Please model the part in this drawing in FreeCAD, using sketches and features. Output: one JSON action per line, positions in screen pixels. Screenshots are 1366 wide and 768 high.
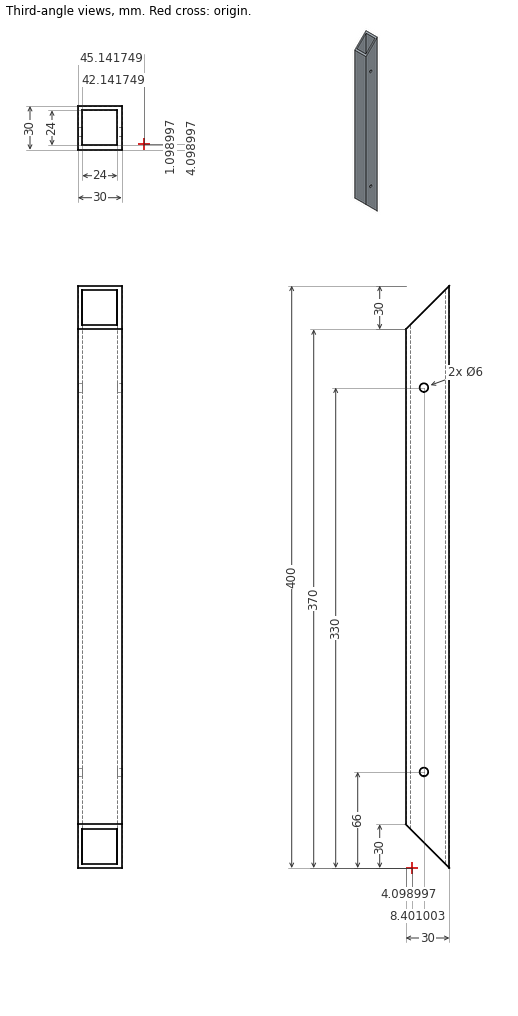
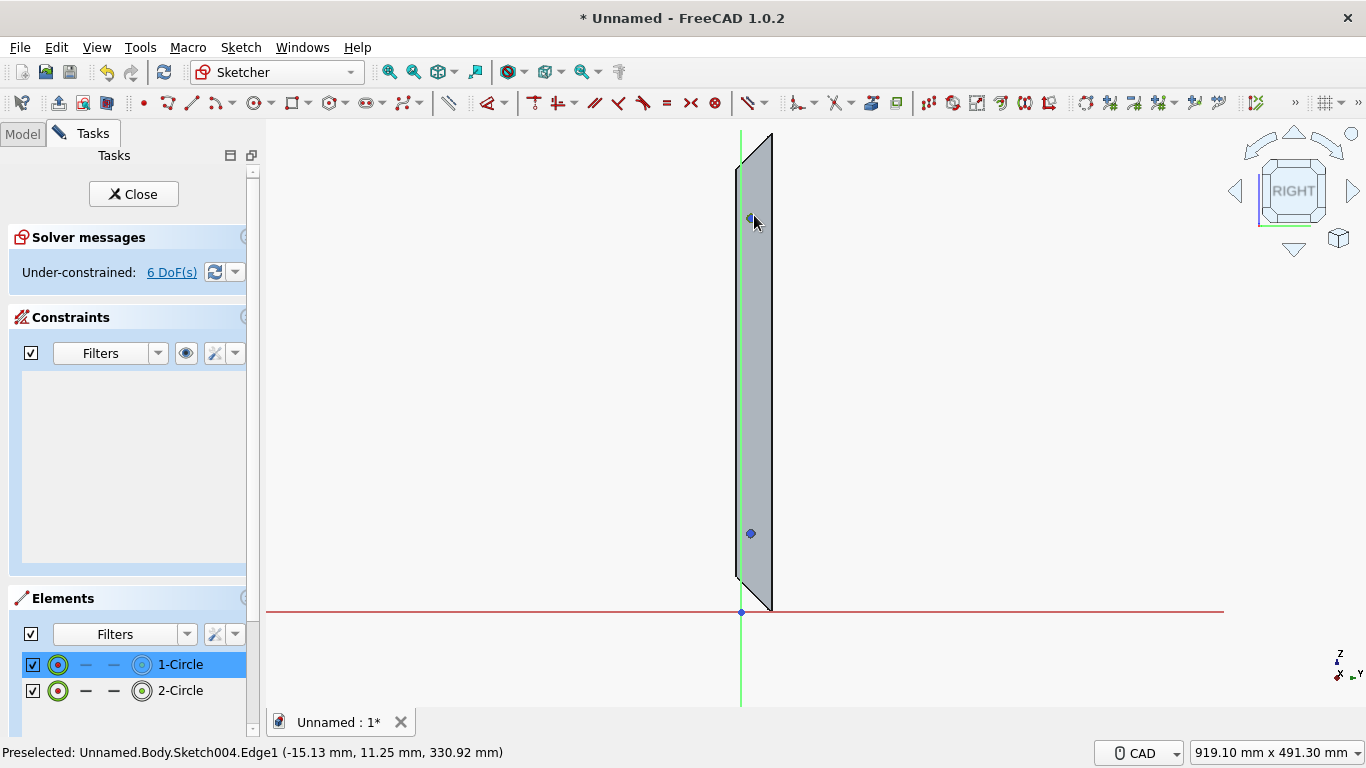
{"action": "scroll", "coordinate": [754, 531], "scroll_direction": "up", "scroll_amount": 7}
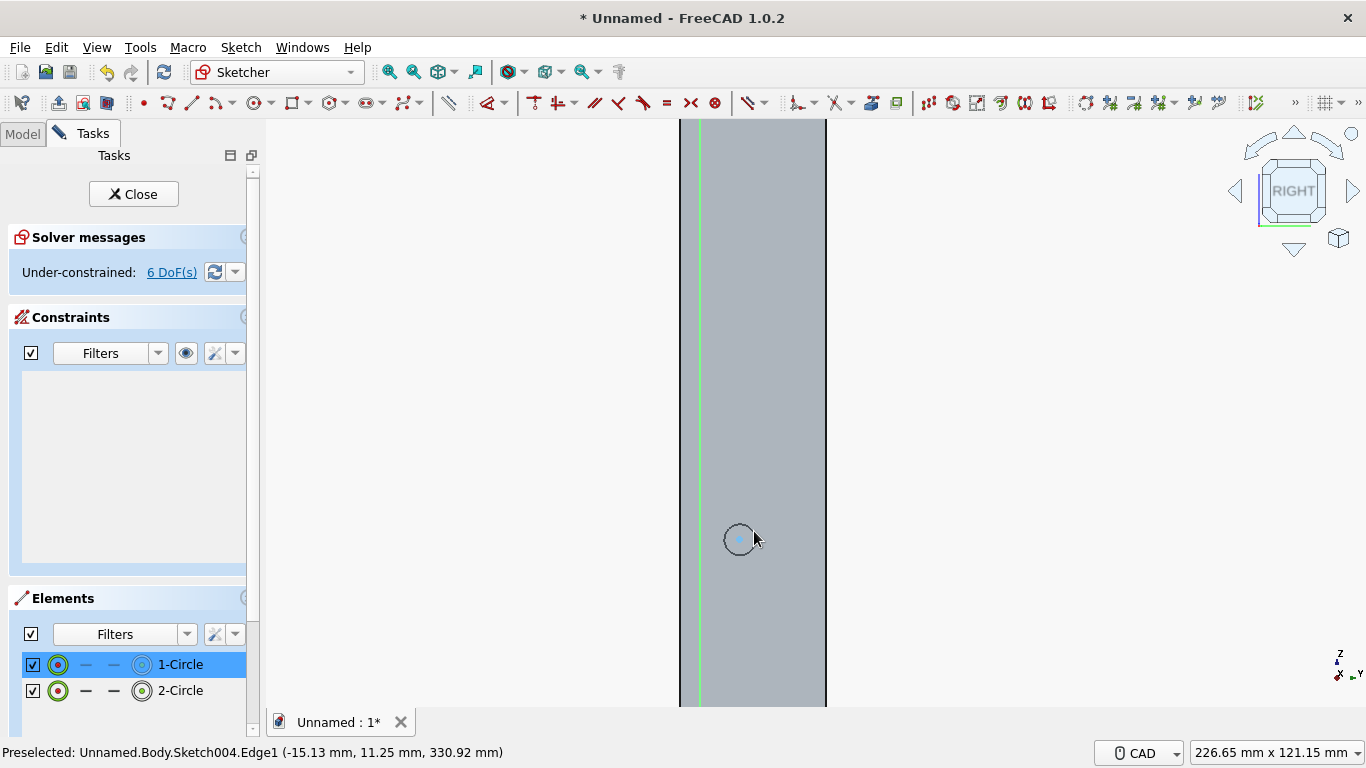
{"action": "left_click", "coordinate": [751, 529]}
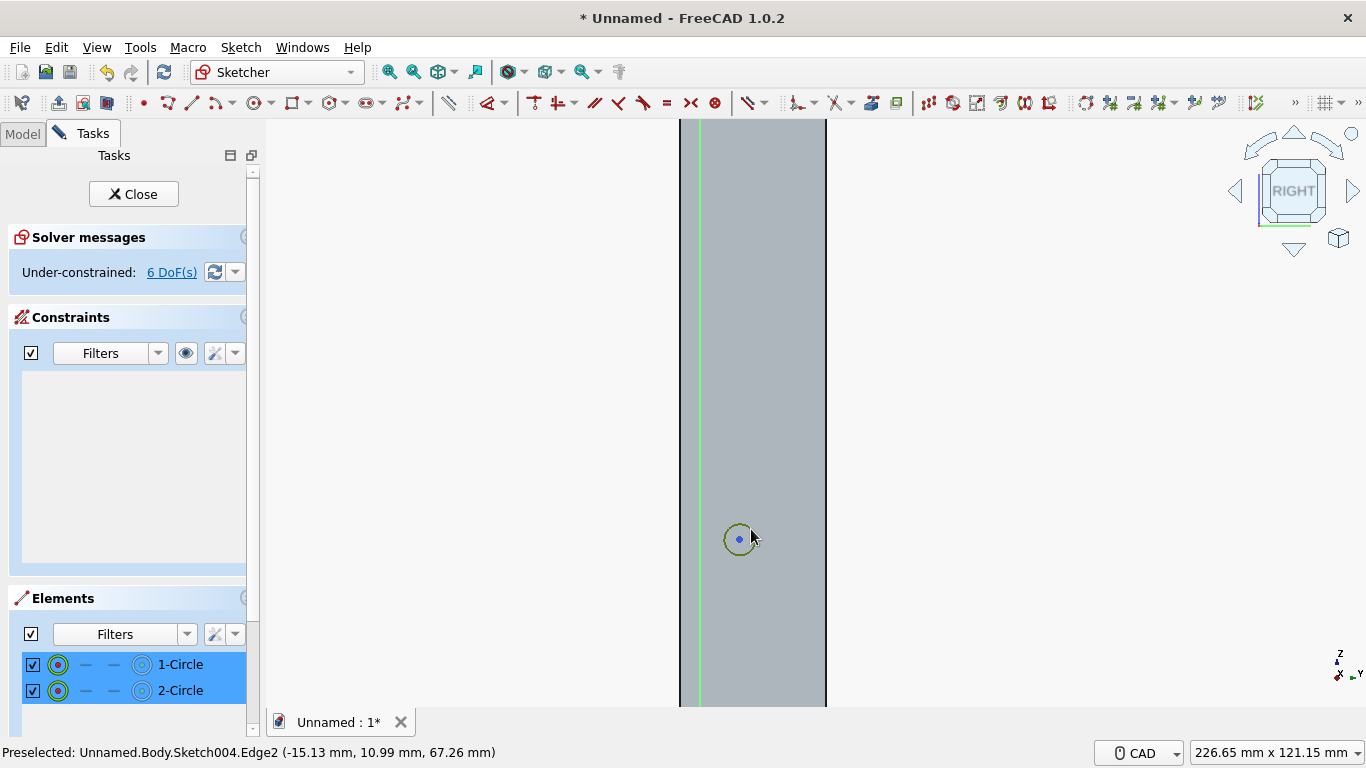
{"action": "left_click", "coordinate": [668, 104]}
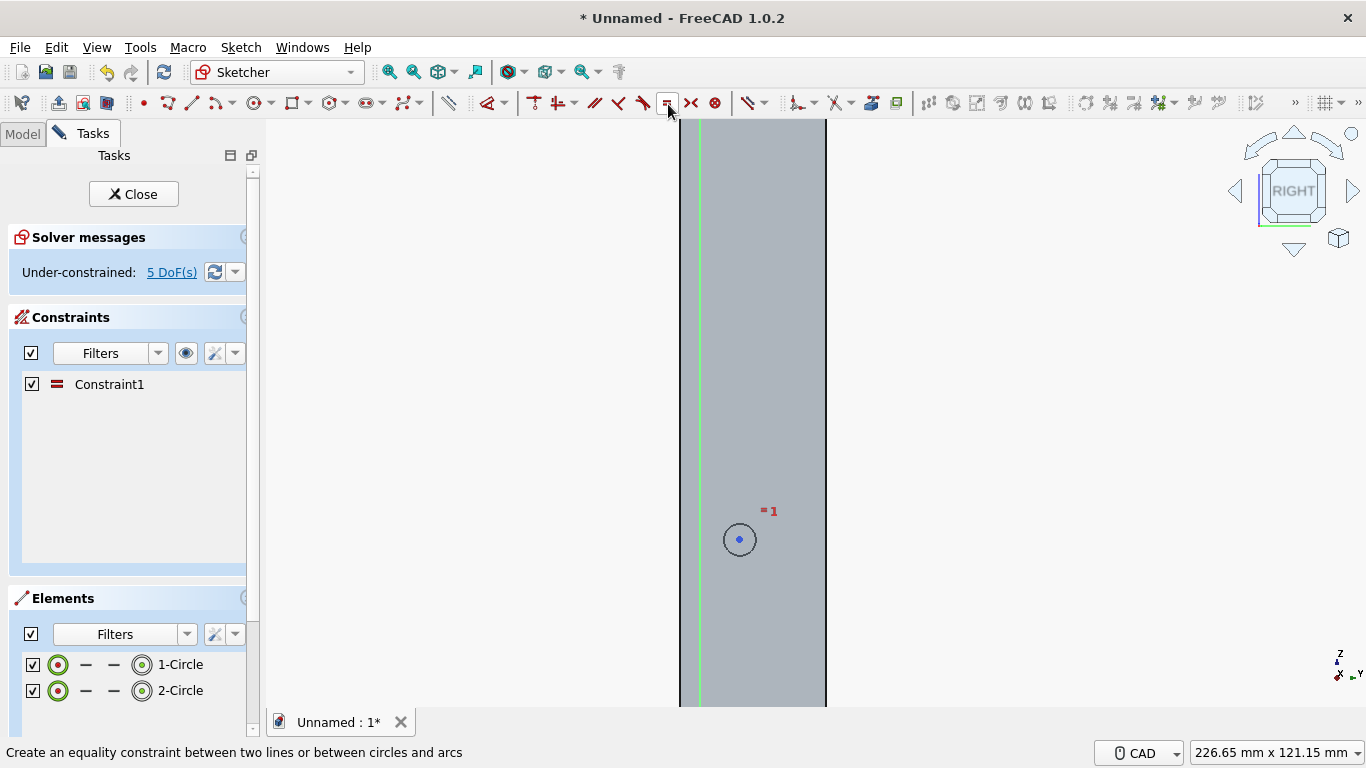
{"action": "scroll", "coordinate": [754, 532], "scroll_direction": "down", "scroll_amount": 7}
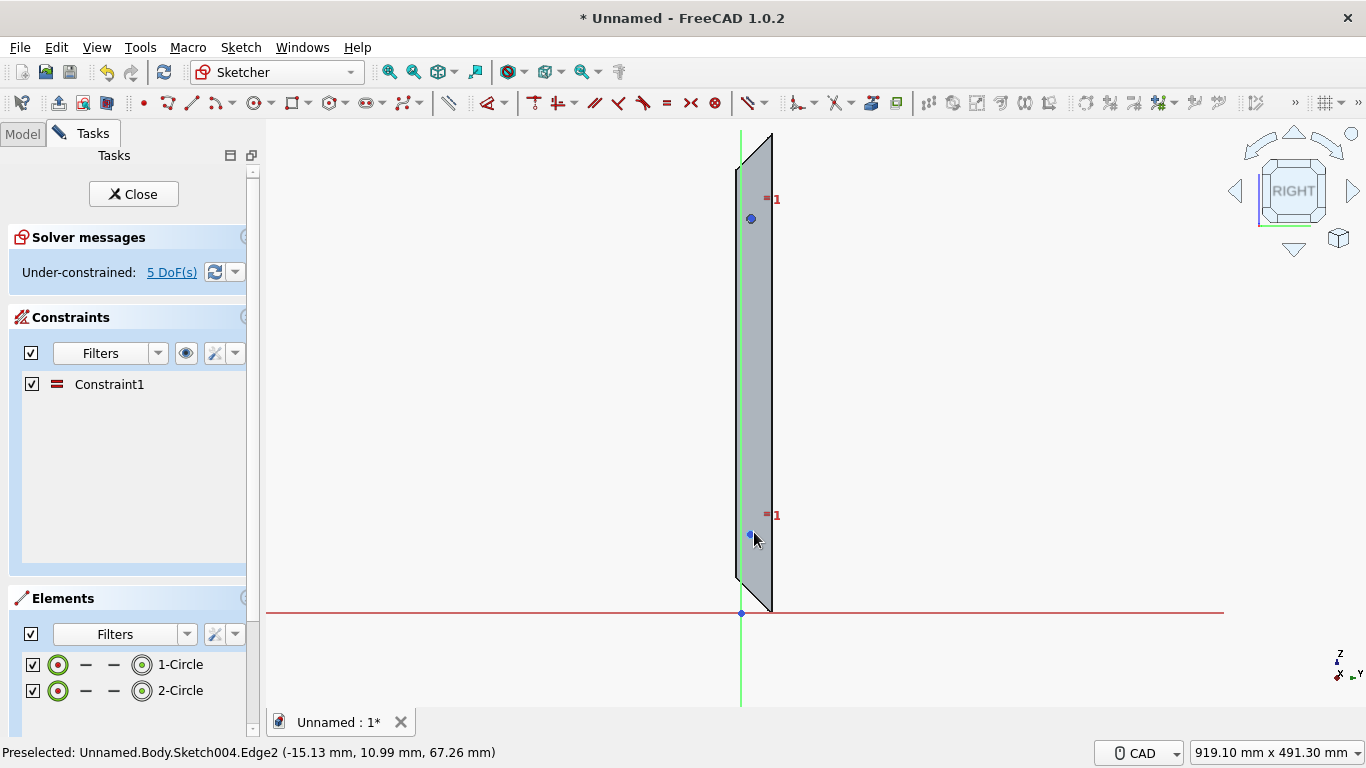
{"action": "left_click", "coordinate": [751, 219]}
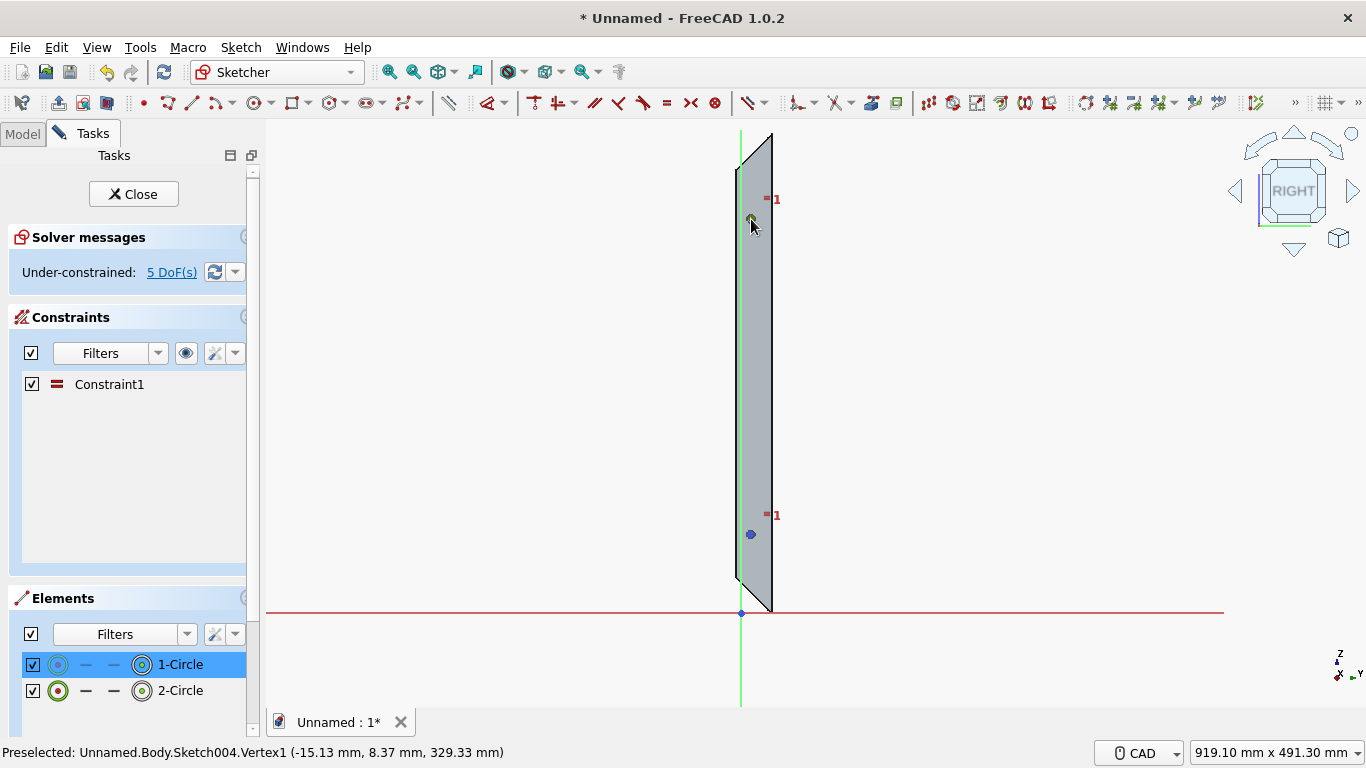
{"action": "left_click", "coordinate": [751, 534]}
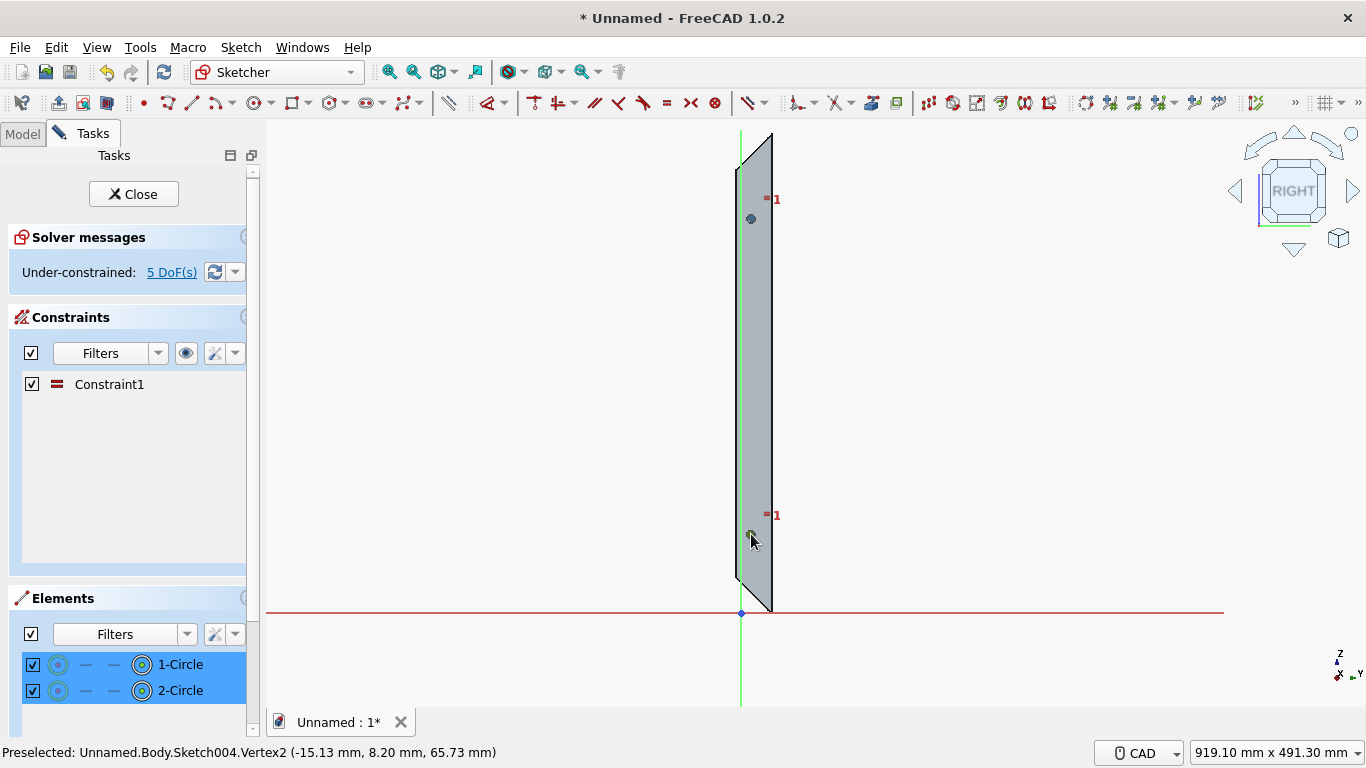
{"action": "left_click", "coordinate": [576, 104]}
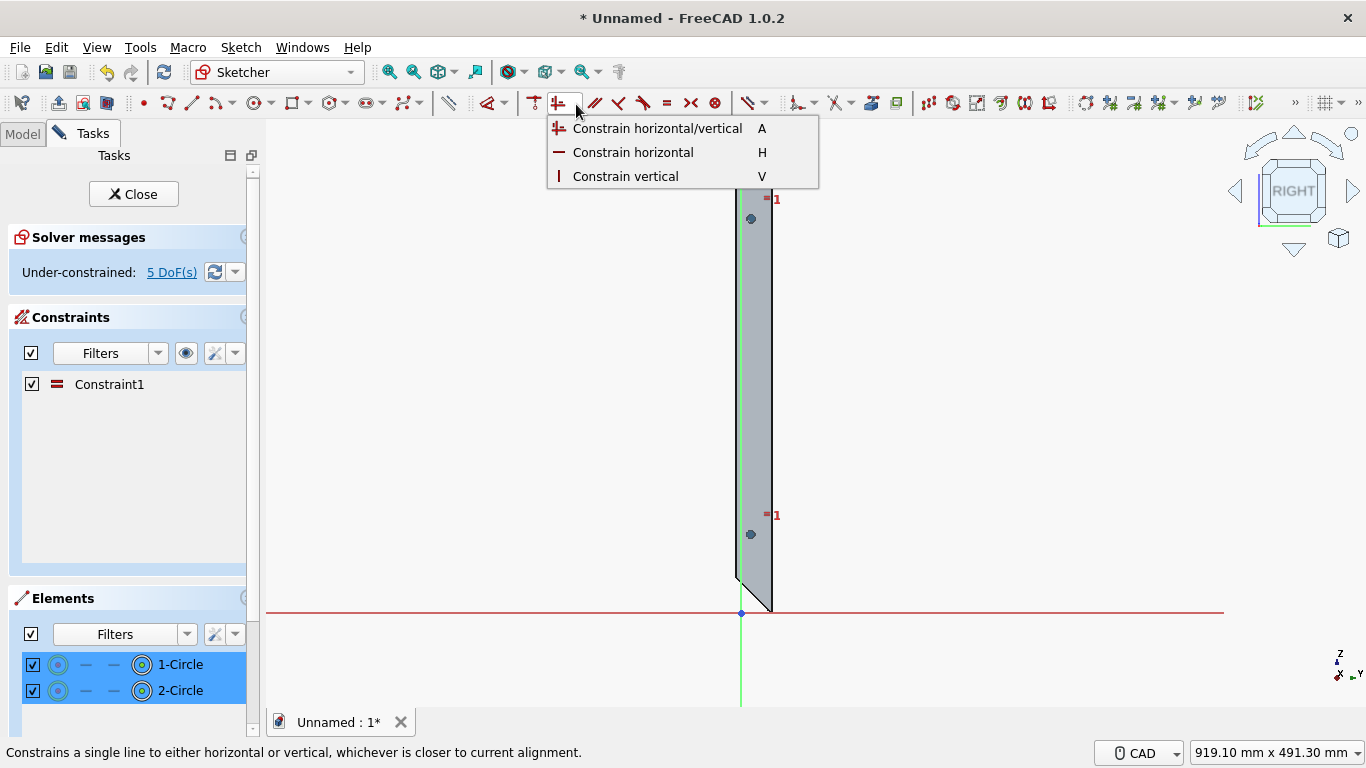
{"action": "left_click", "coordinate": [683, 176]}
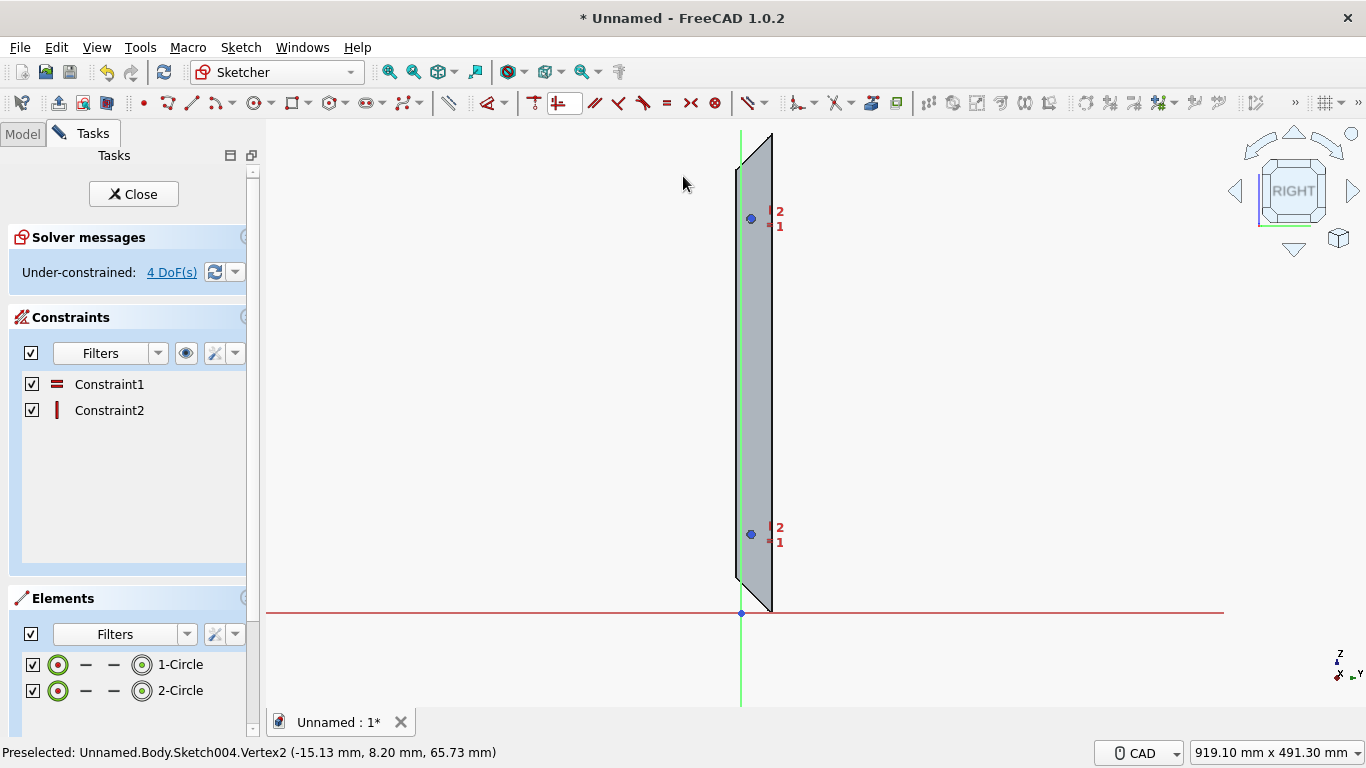
{"action": "key", "text": "d"}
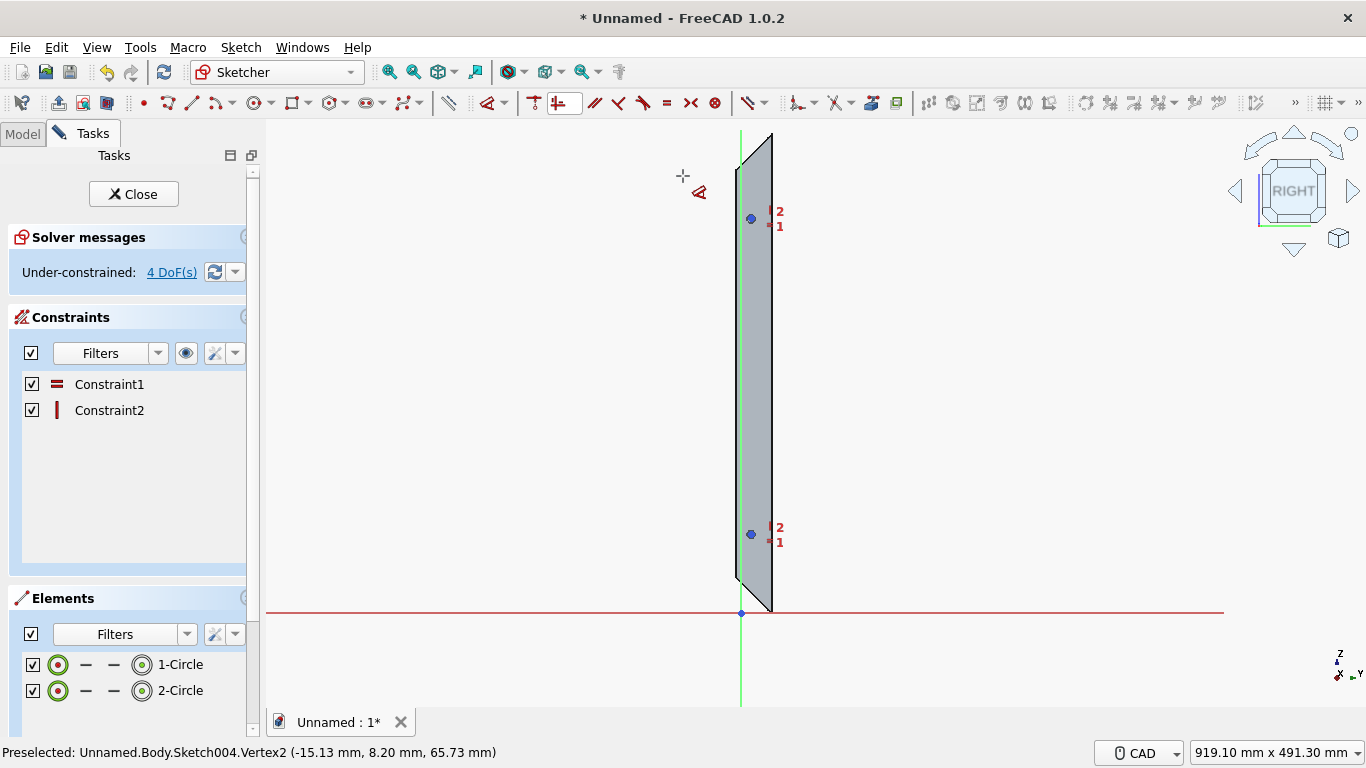
{"action": "scroll", "coordinate": [751, 215], "scroll_direction": "up", "scroll_amount": 9}